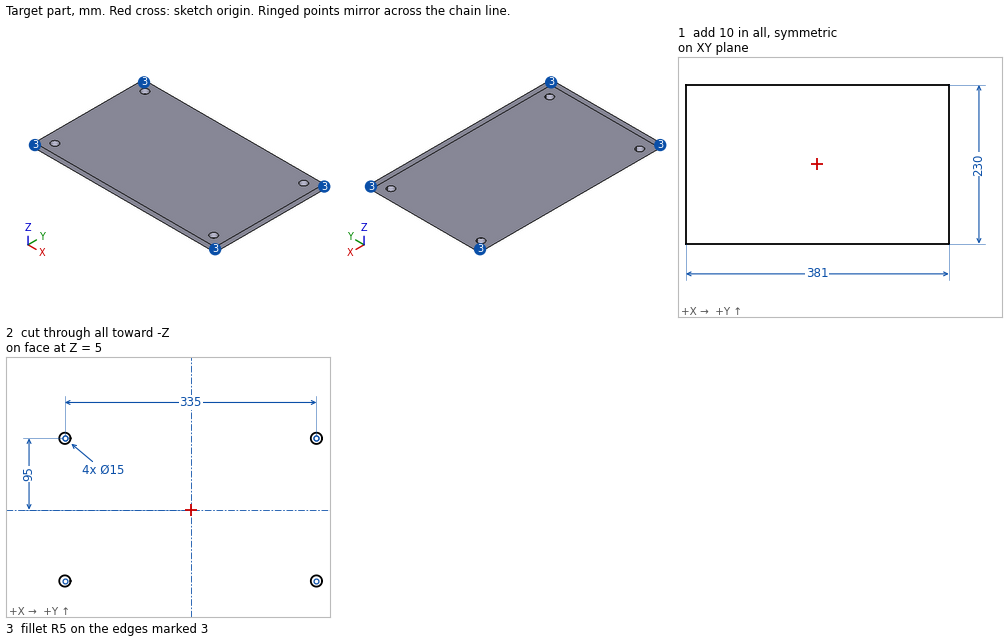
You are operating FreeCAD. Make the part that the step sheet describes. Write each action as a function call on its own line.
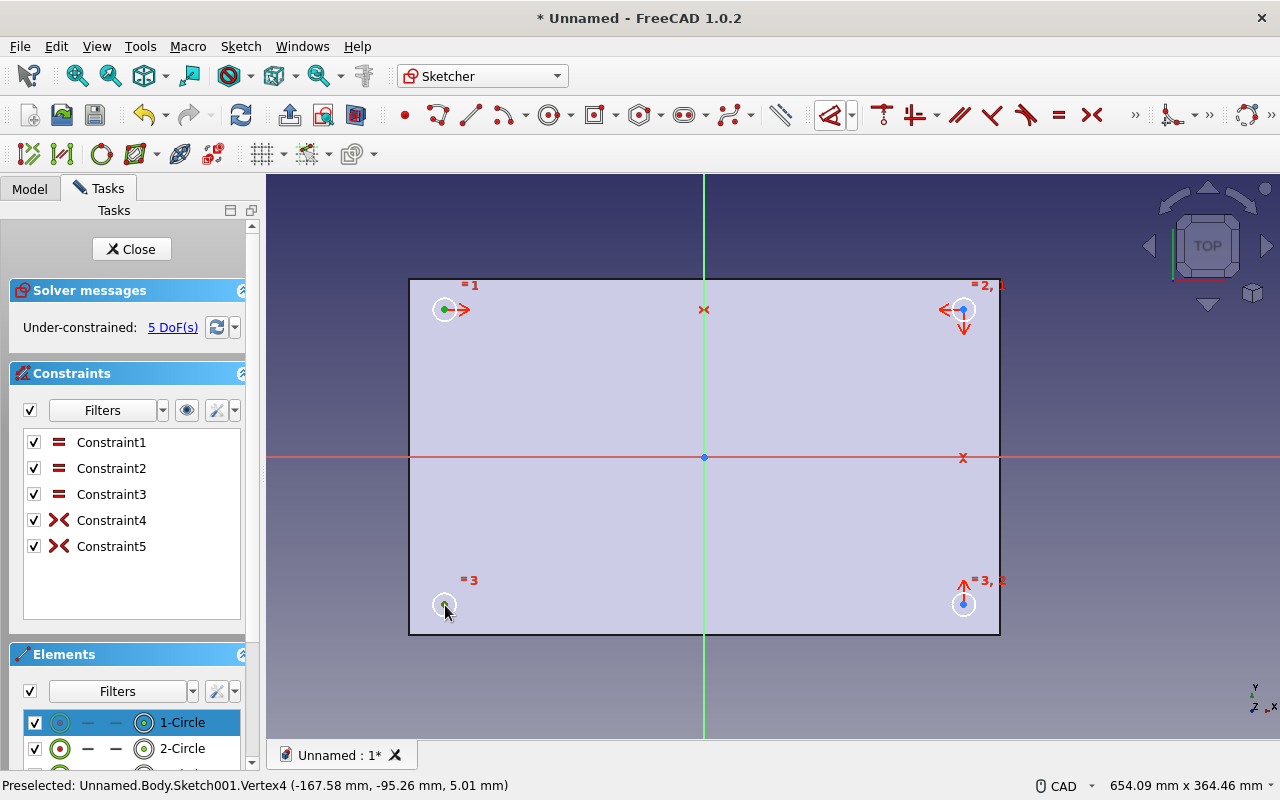
click(353, 457)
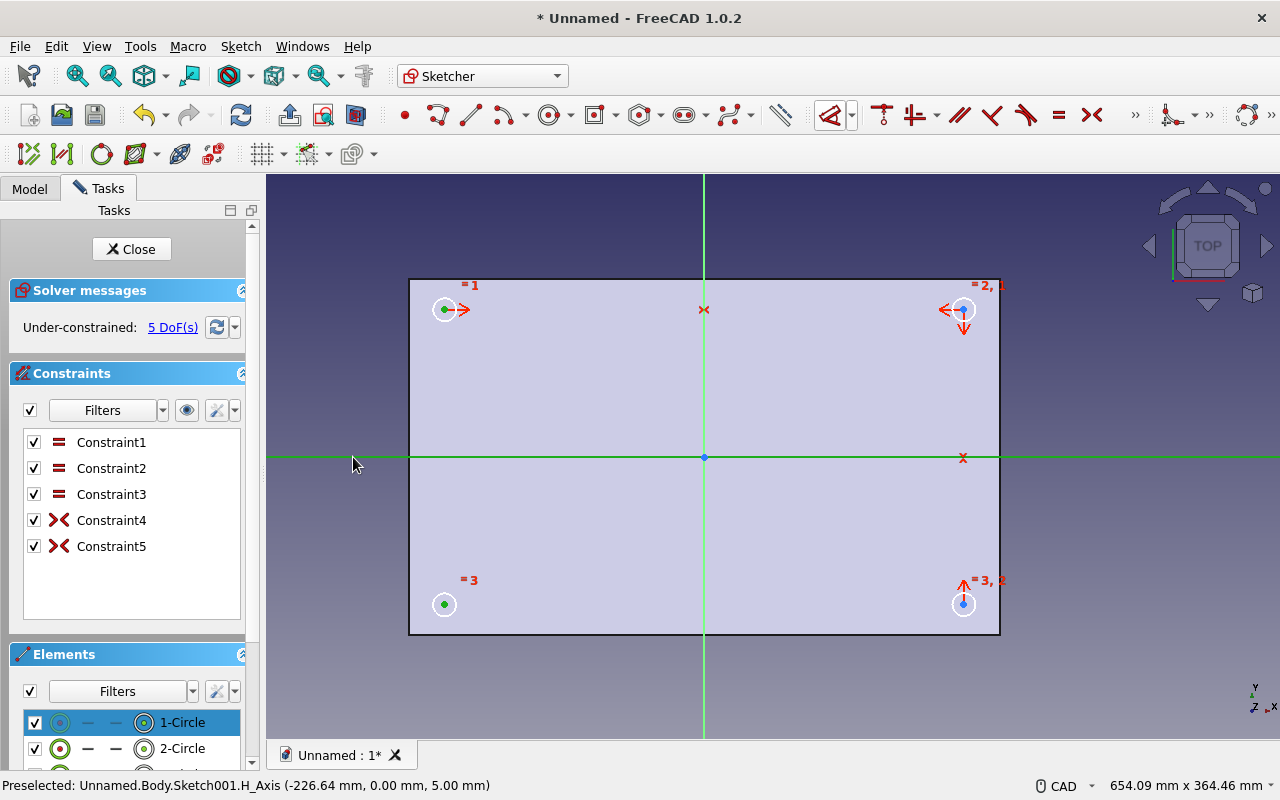
click(1092, 116)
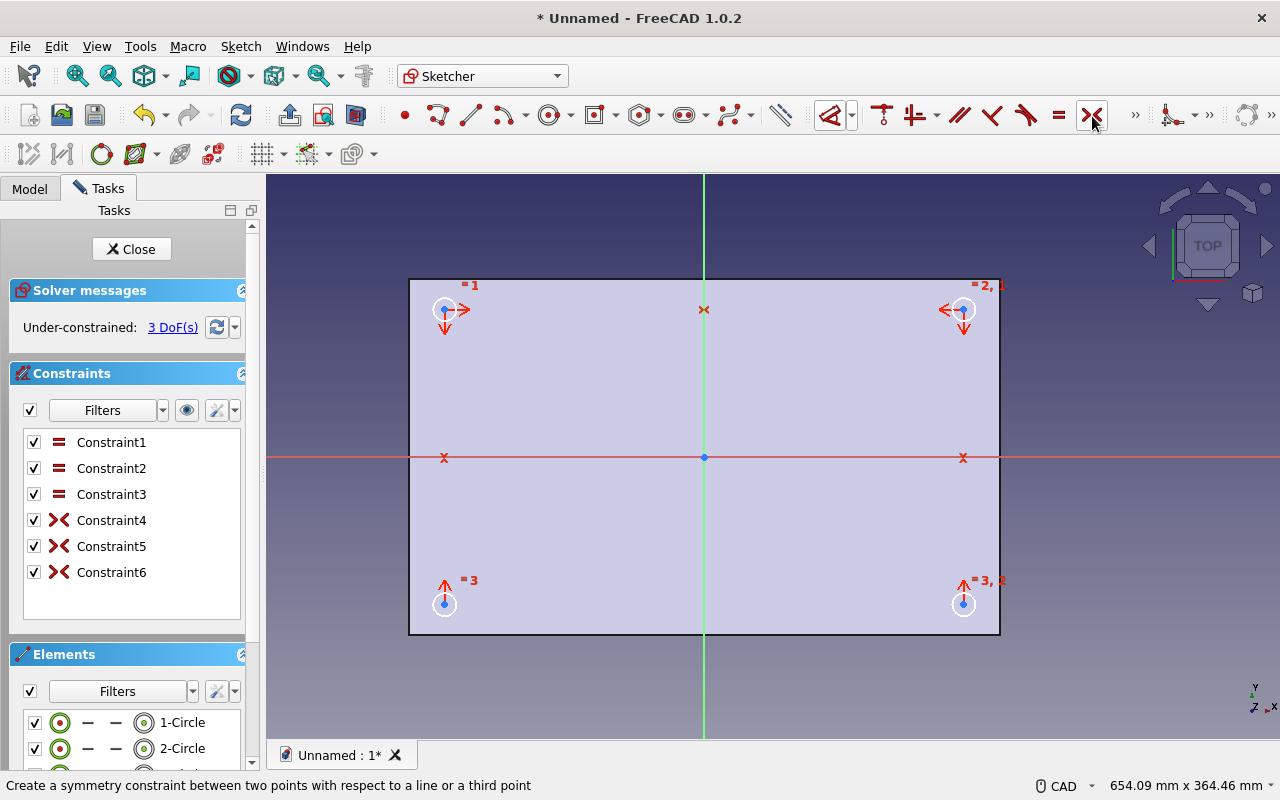
scroll(453, 302, up, 3)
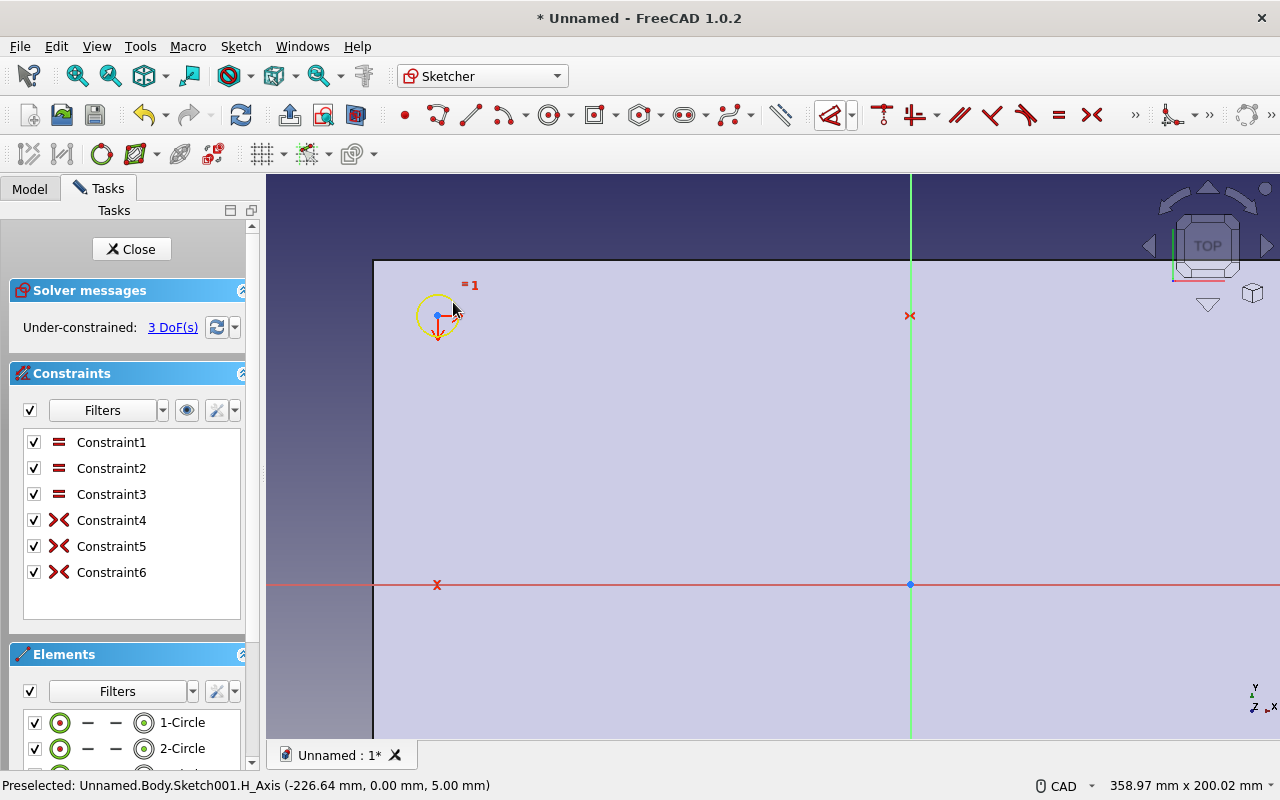
click(453, 301)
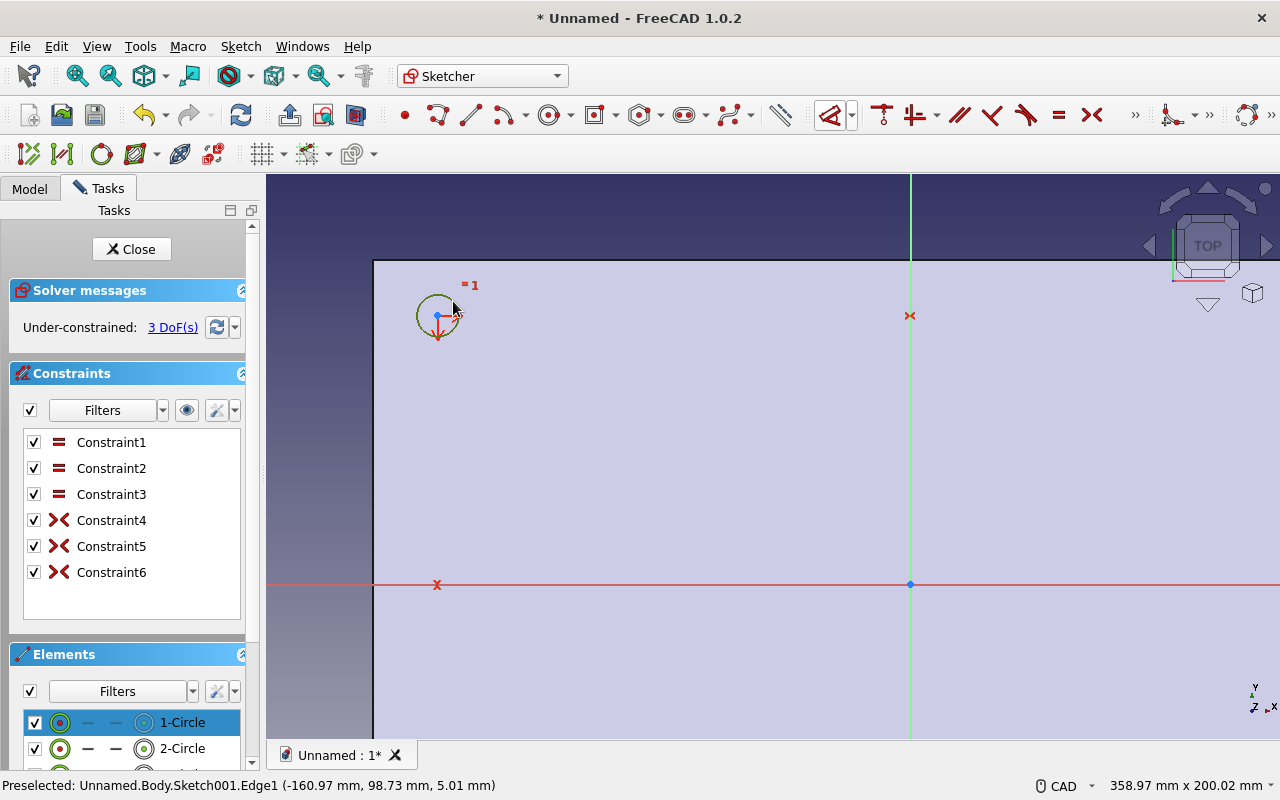
key(k)
key(o)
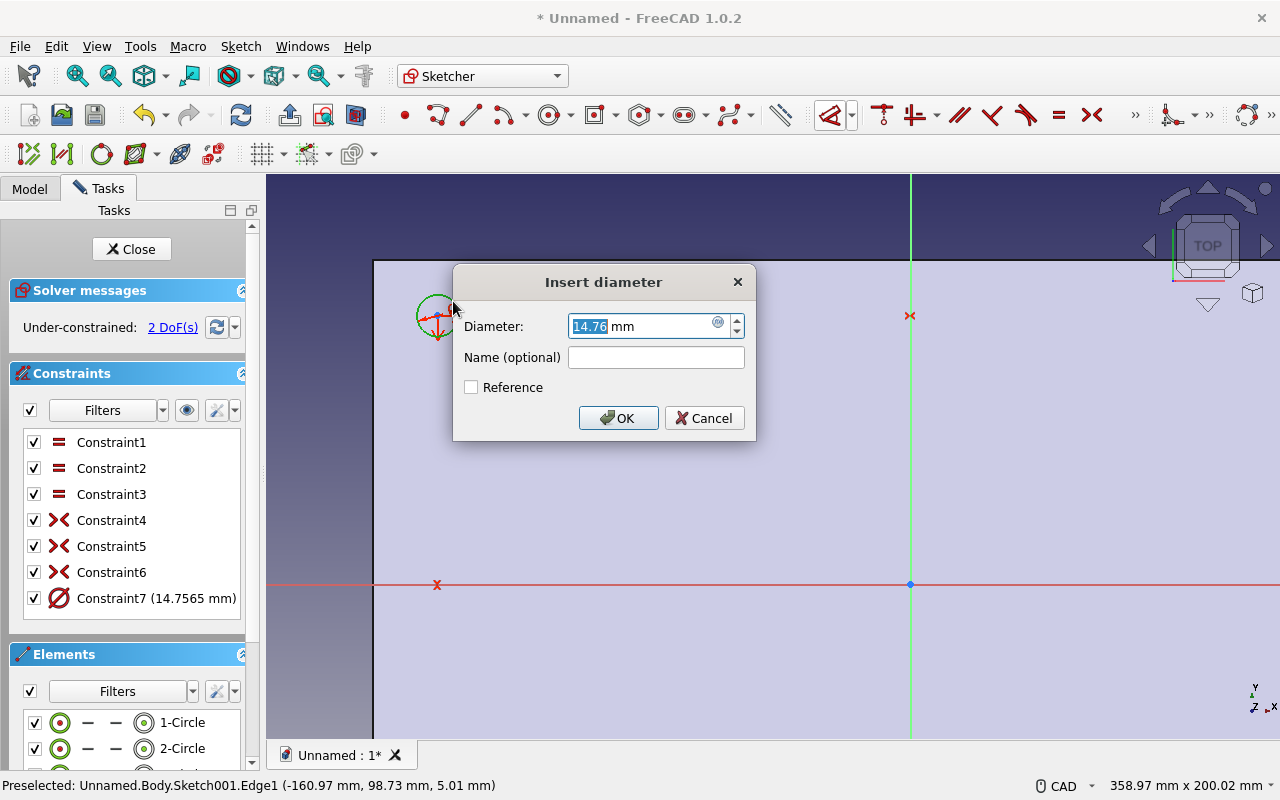
text(15)
key(Return)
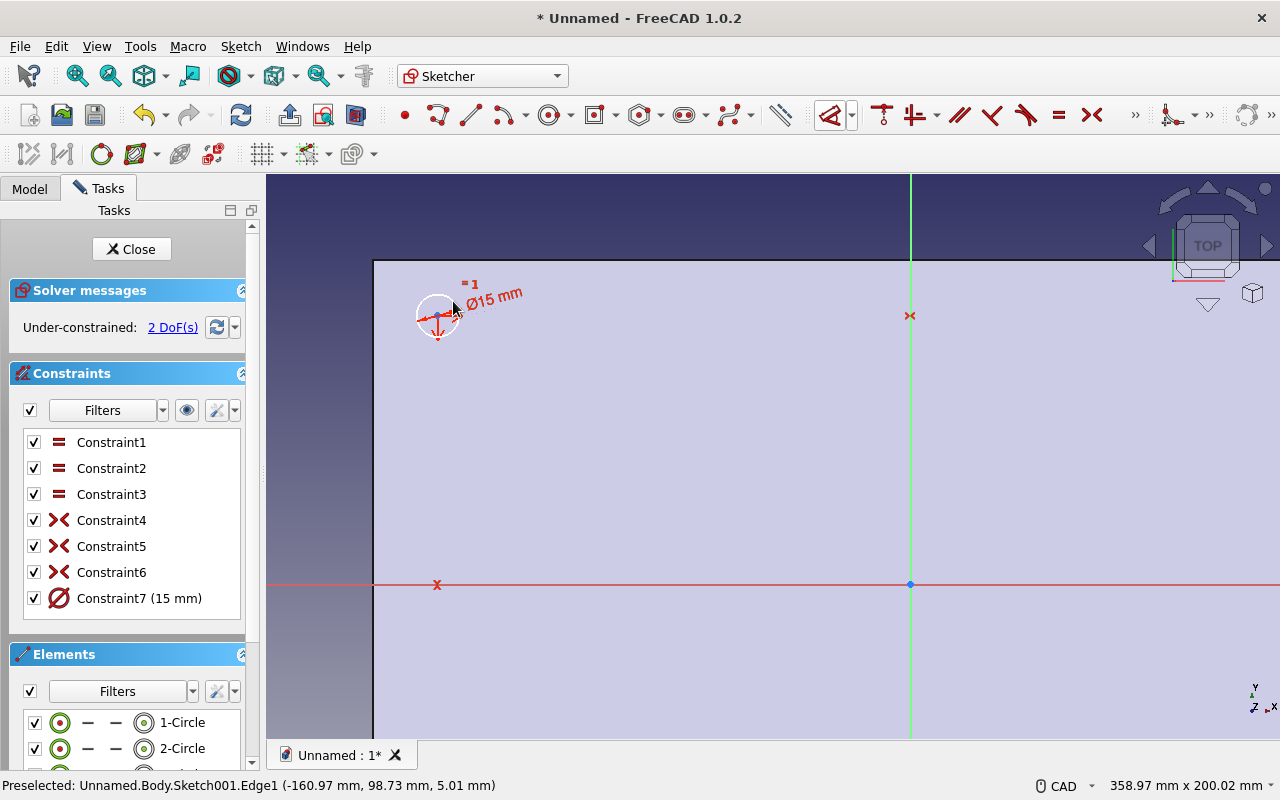
click(438, 316)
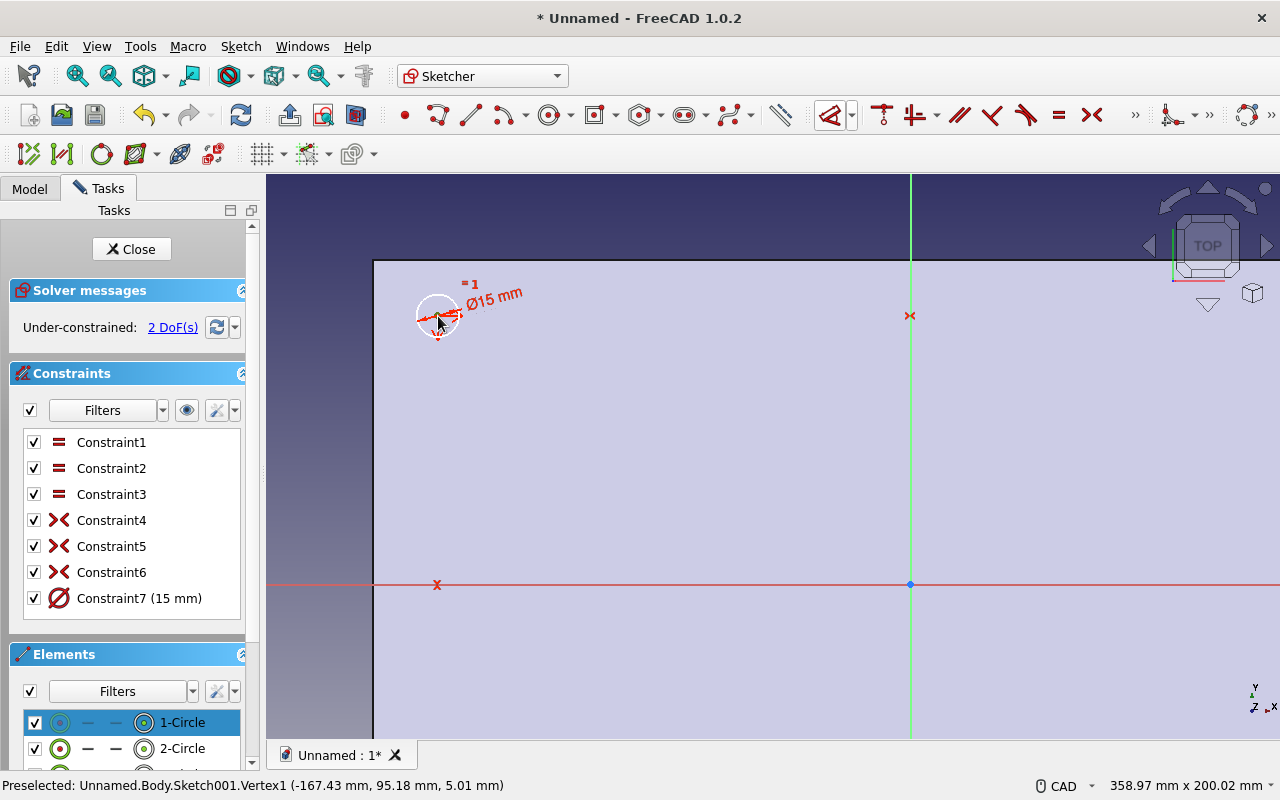
key(i)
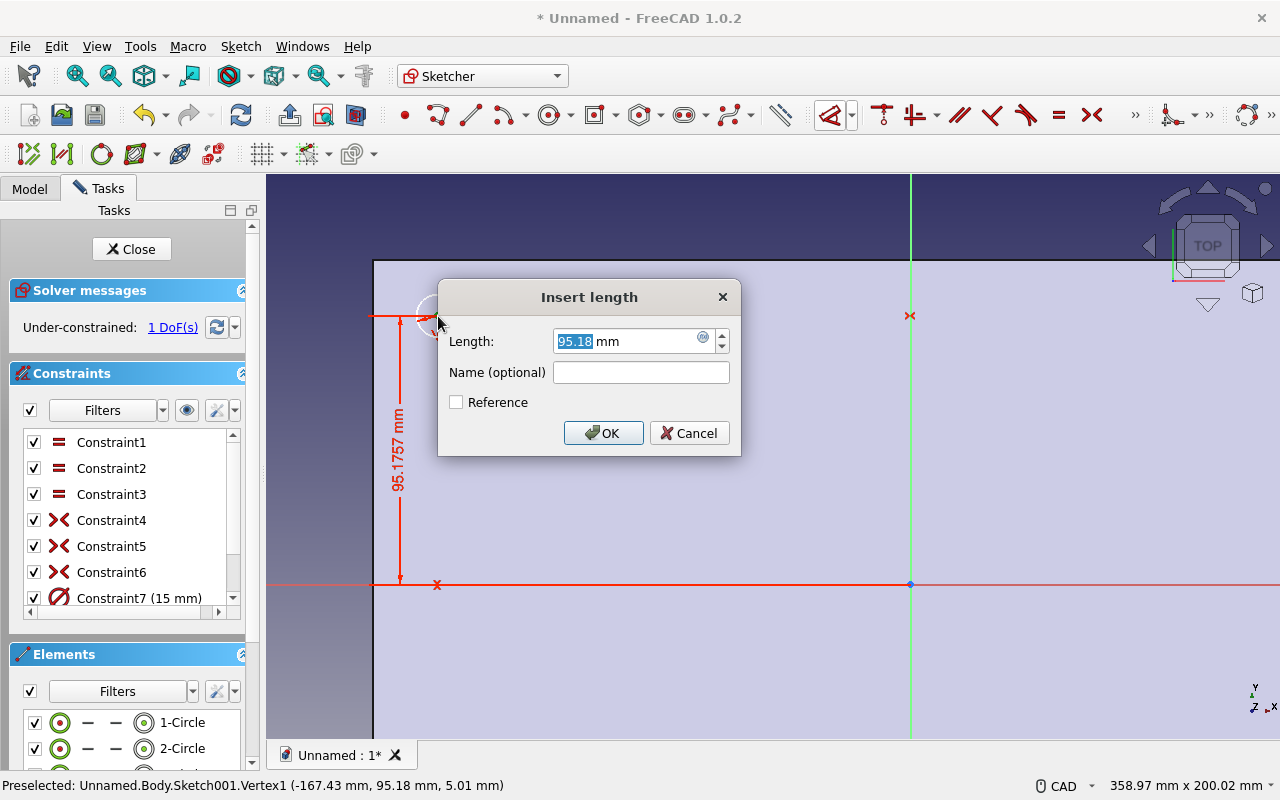
text(95)
key(Return)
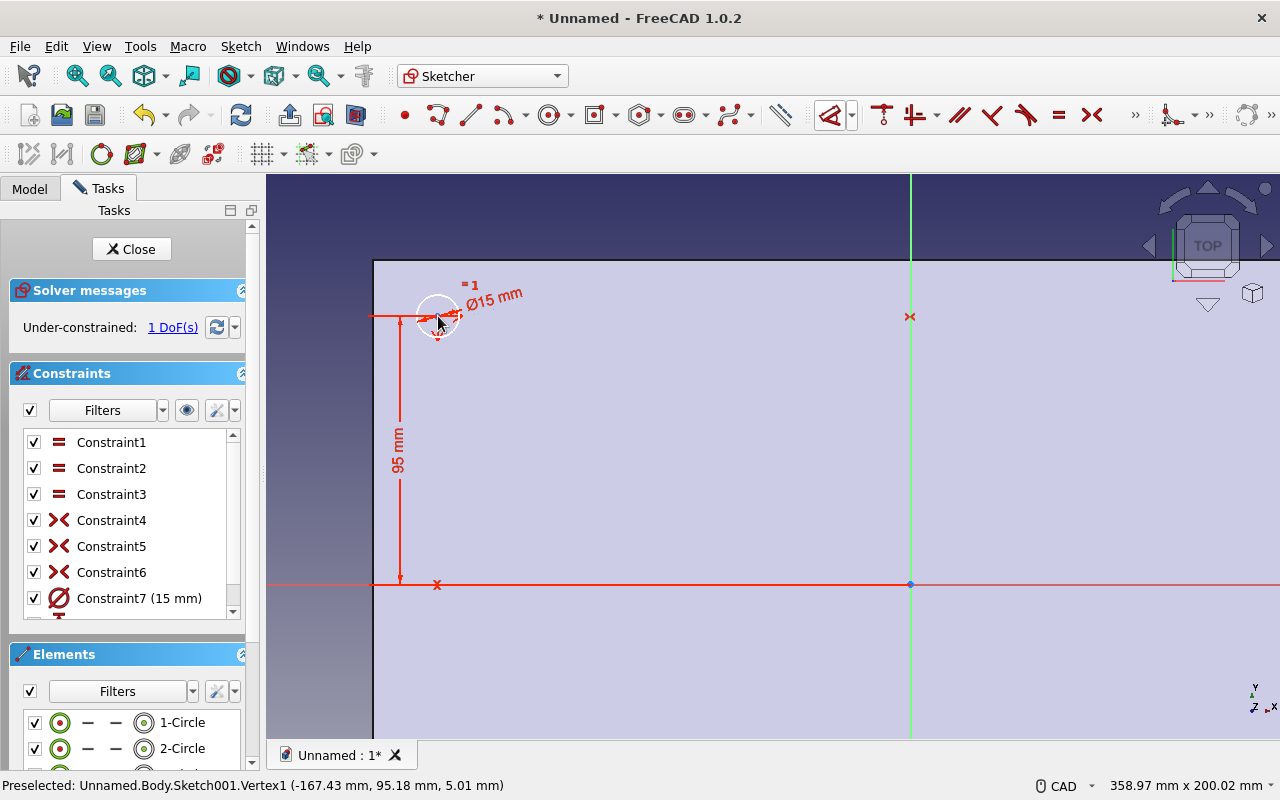
click(438, 316)